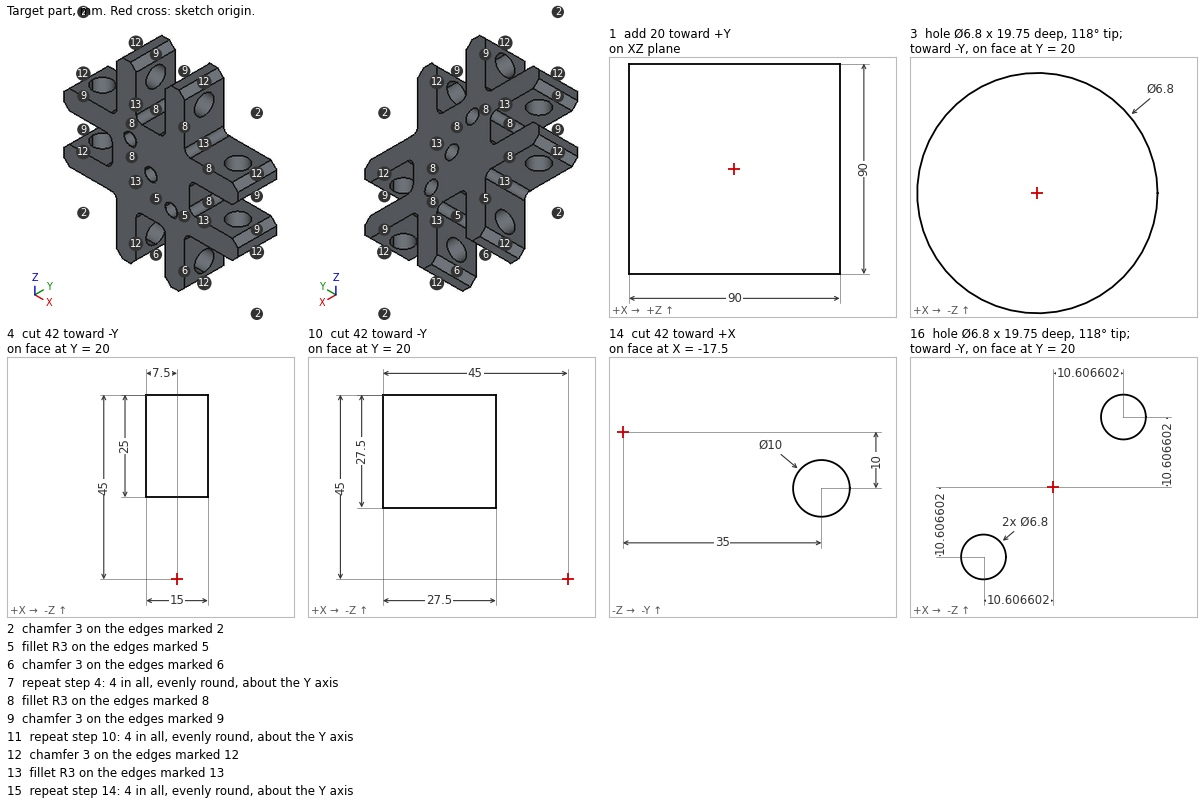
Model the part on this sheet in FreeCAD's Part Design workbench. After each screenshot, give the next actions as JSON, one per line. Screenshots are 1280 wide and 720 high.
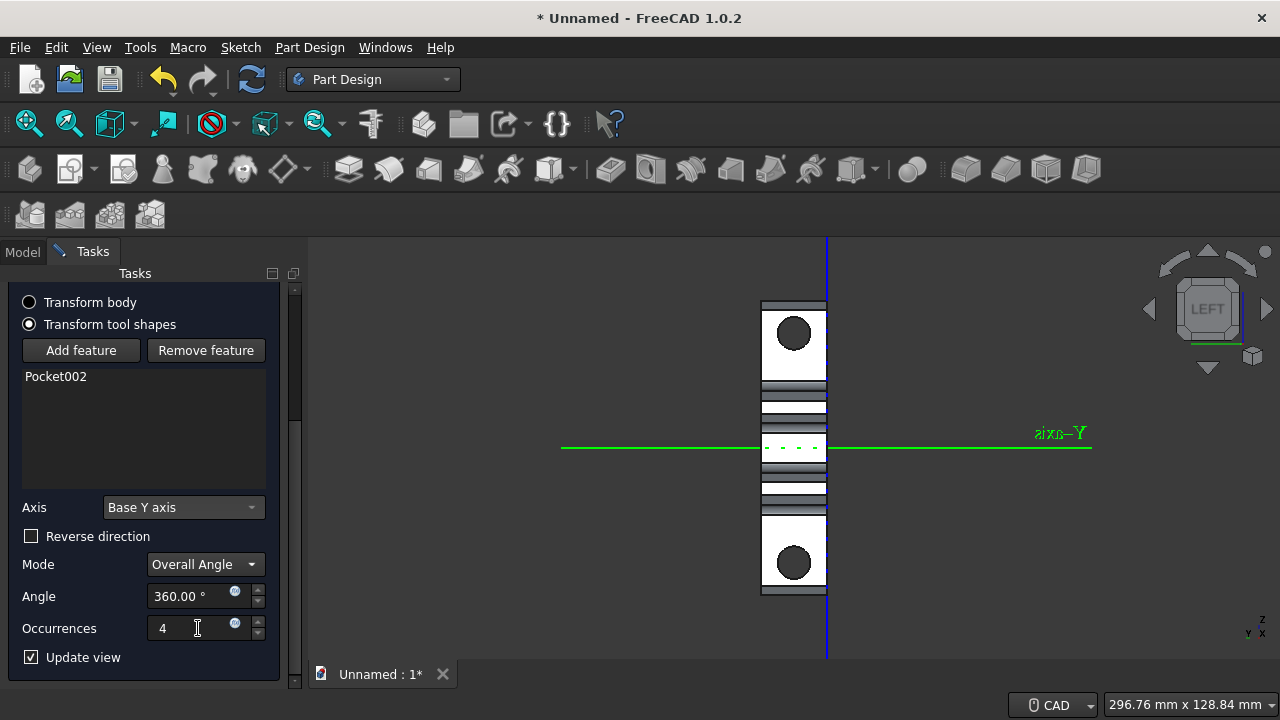
{"action": "scroll", "coordinate": [295, 486], "scroll_direction": "up", "scroll_amount": 5}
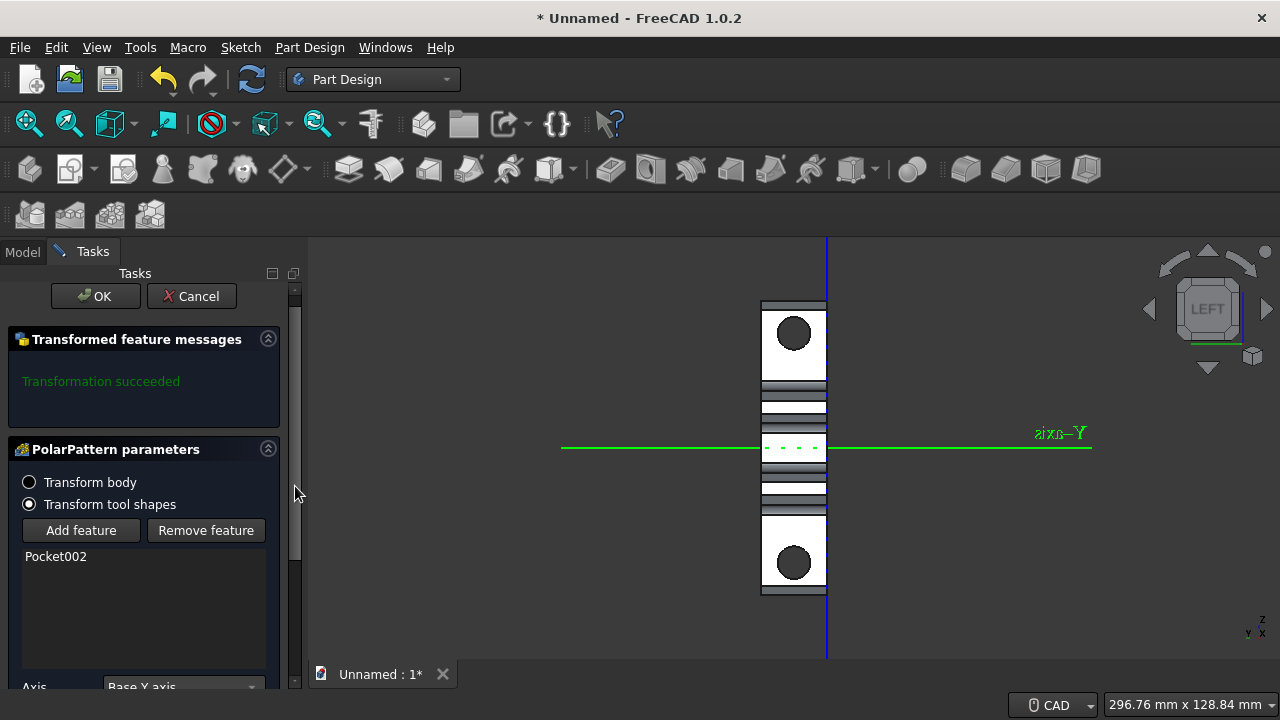
{"action": "left_click", "coordinate": [96, 312]}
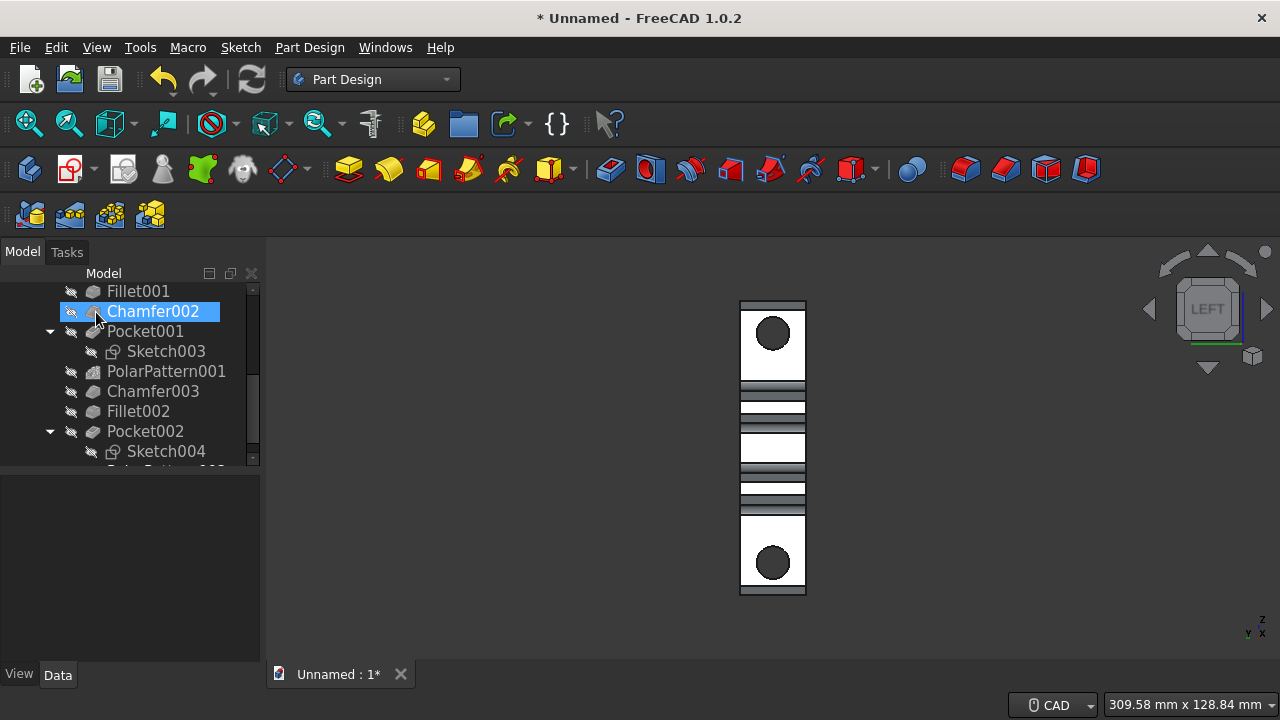
{"action": "key", "text": "4"}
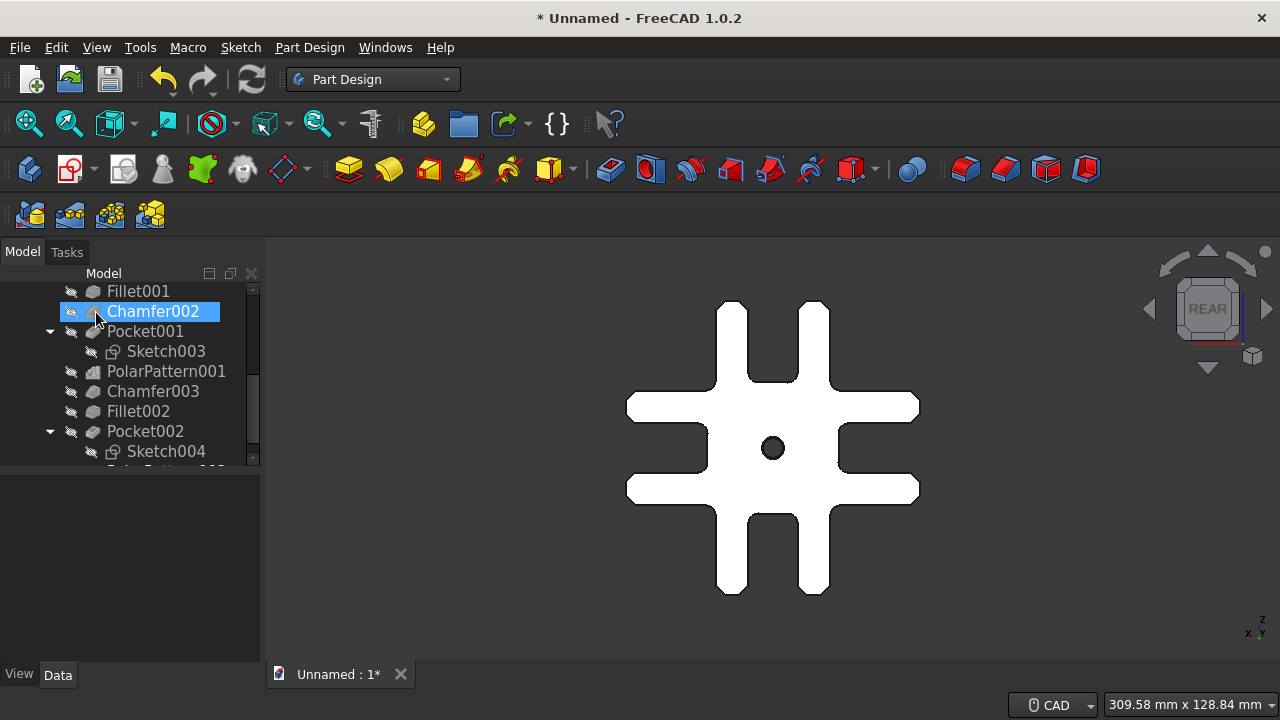
{"action": "left_click", "coordinate": [731, 405]}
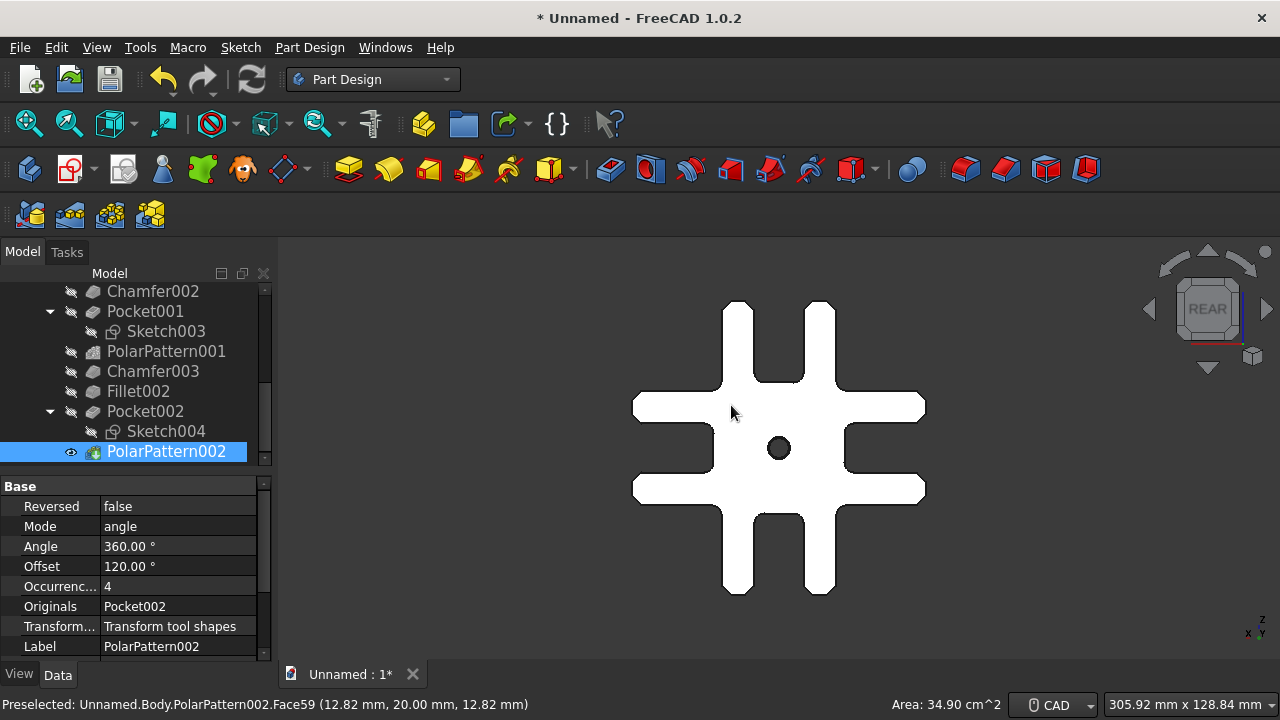
{"action": "left_click", "coordinate": [70, 170]}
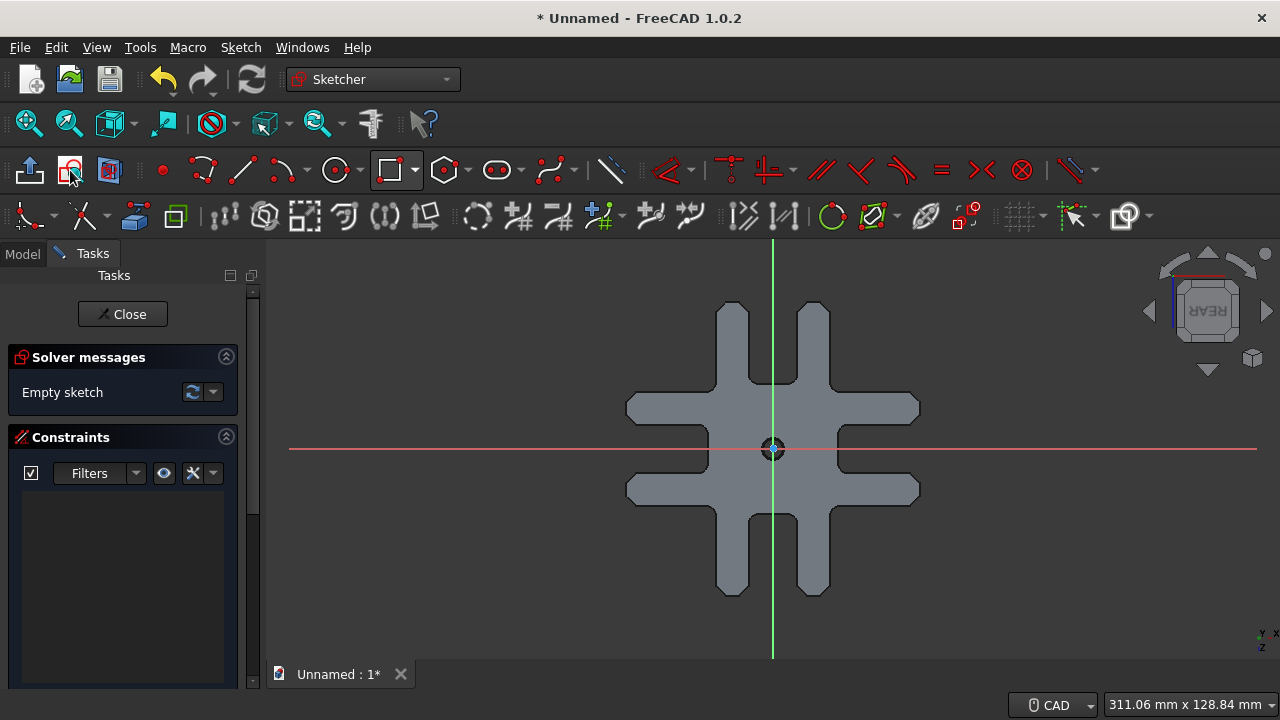
{"action": "scroll", "coordinate": [813, 449], "scroll_direction": "up", "scroll_amount": 5}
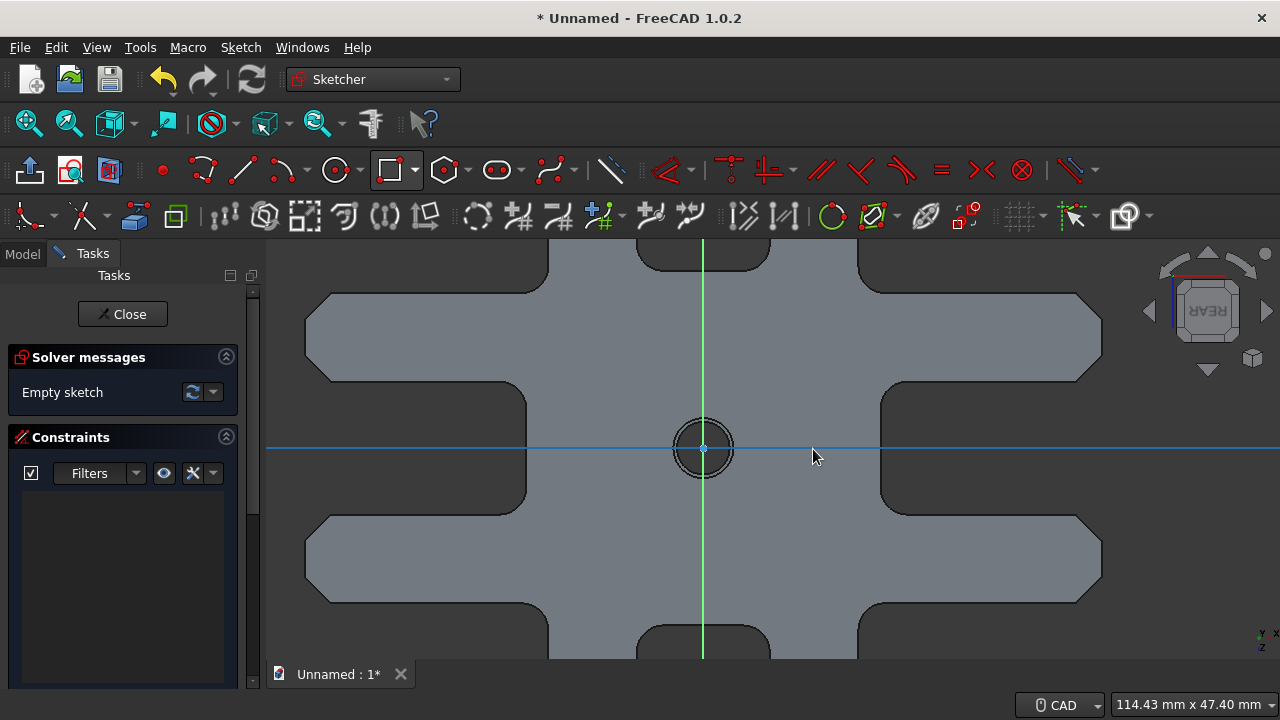
{"action": "left_click", "coordinate": [336, 170]}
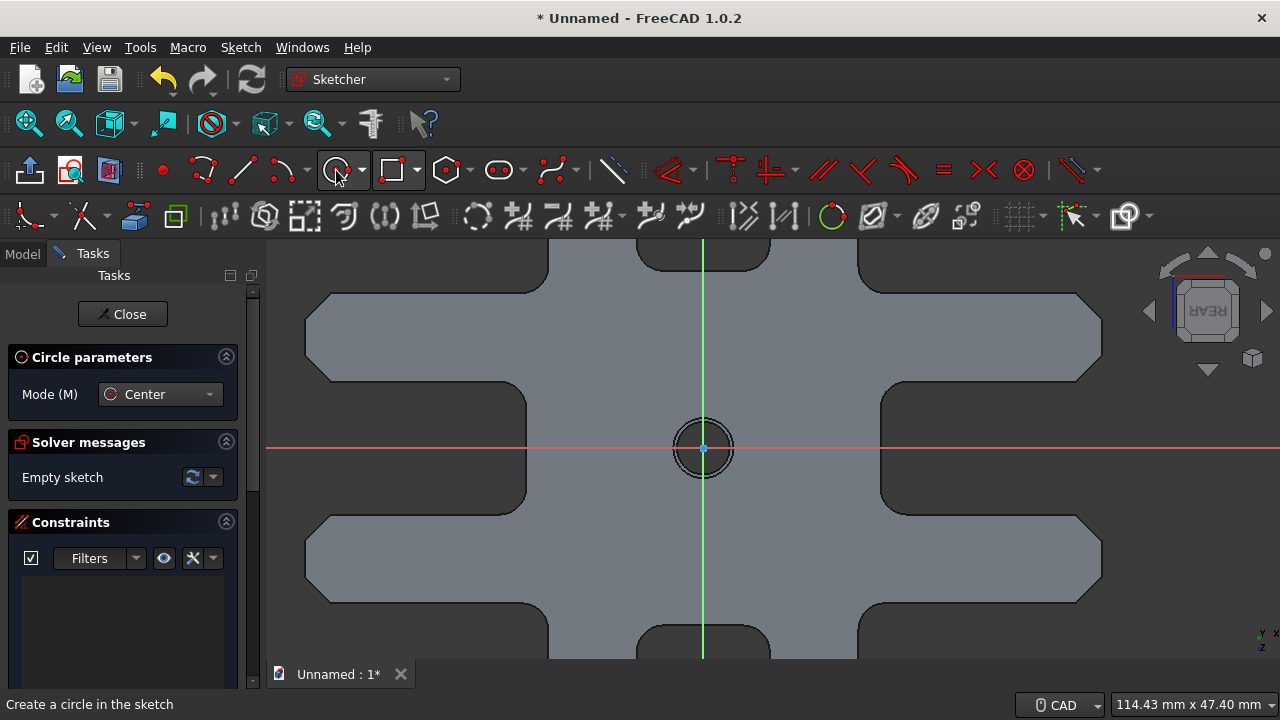
{"action": "left_click", "coordinate": [609, 542]}
{"action": "left_click", "coordinate": [631, 521]}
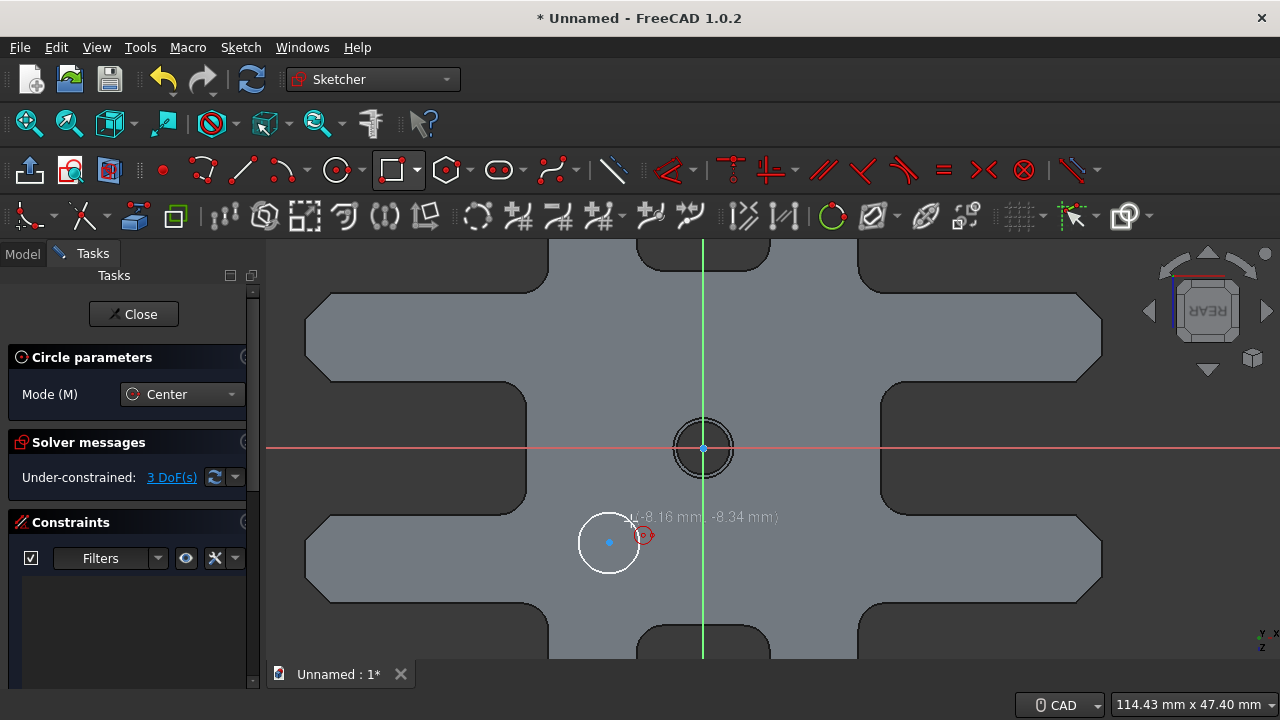
{"action": "left_click", "coordinate": [797, 354]}
{"action": "left_click", "coordinate": [819, 333]}
{"action": "key", "text": "Escape"}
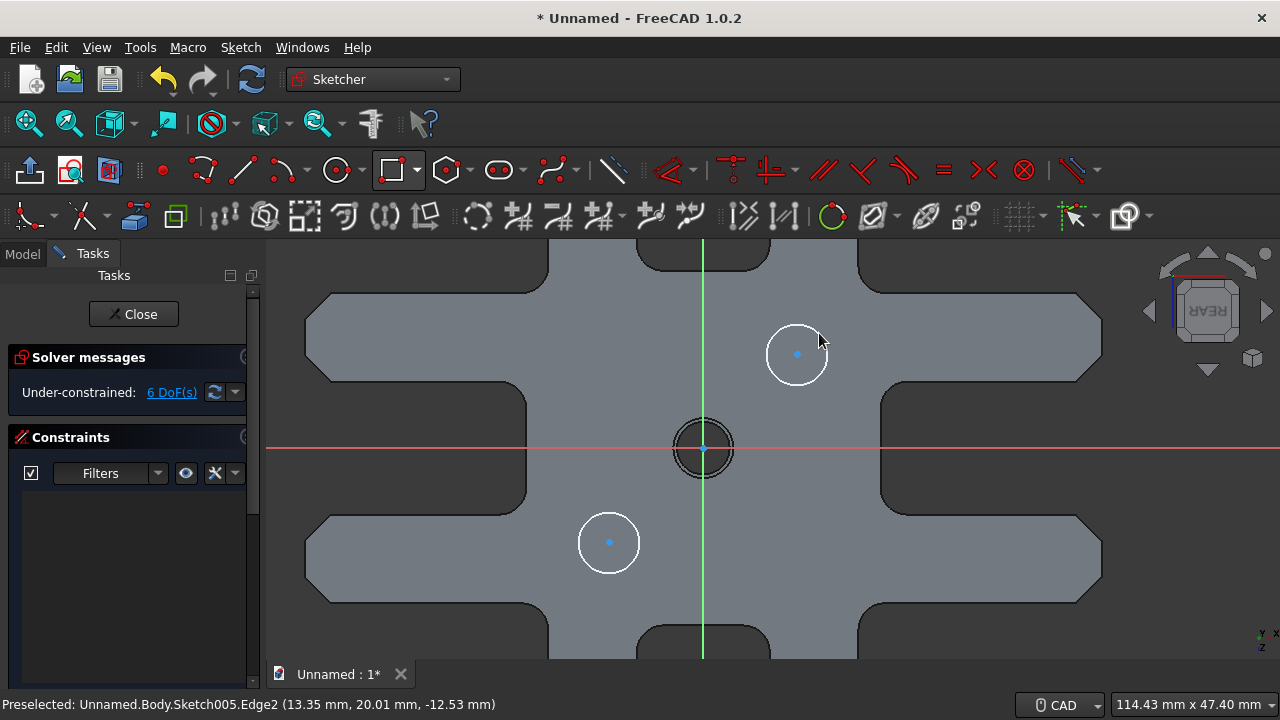
{"action": "left_click", "coordinate": [630, 521]}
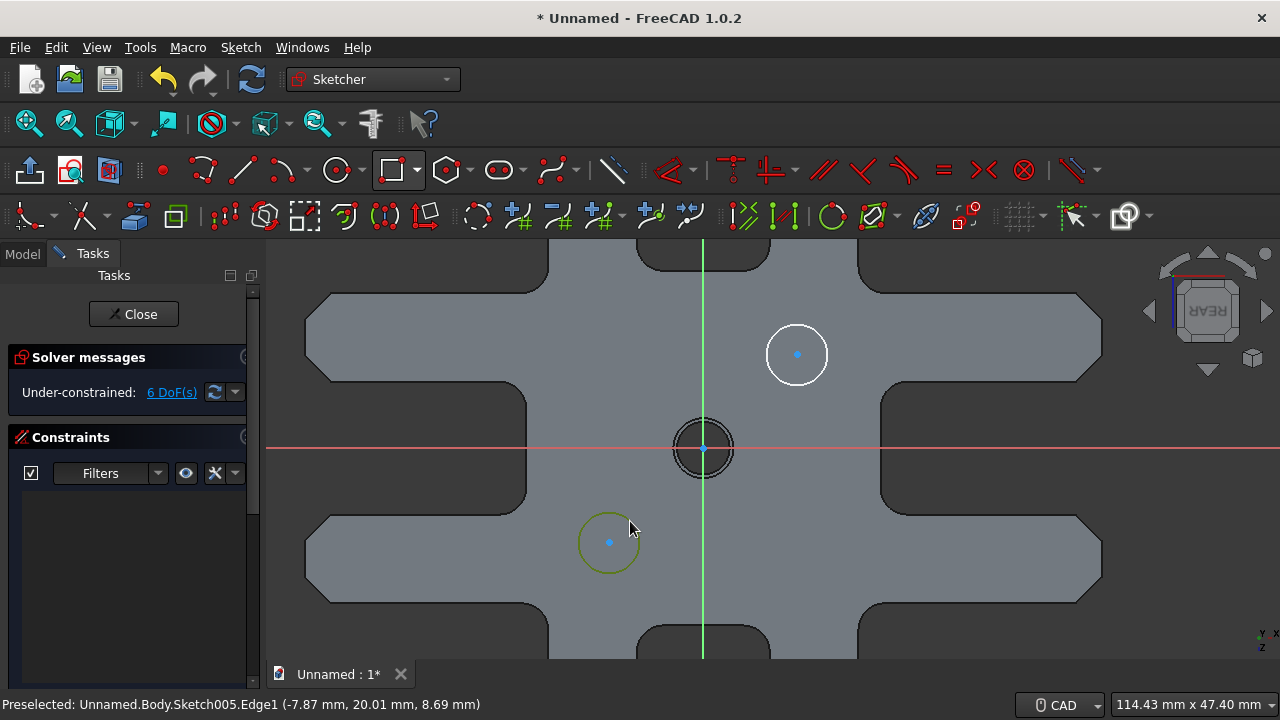
{"action": "left_click", "coordinate": [818, 333]}